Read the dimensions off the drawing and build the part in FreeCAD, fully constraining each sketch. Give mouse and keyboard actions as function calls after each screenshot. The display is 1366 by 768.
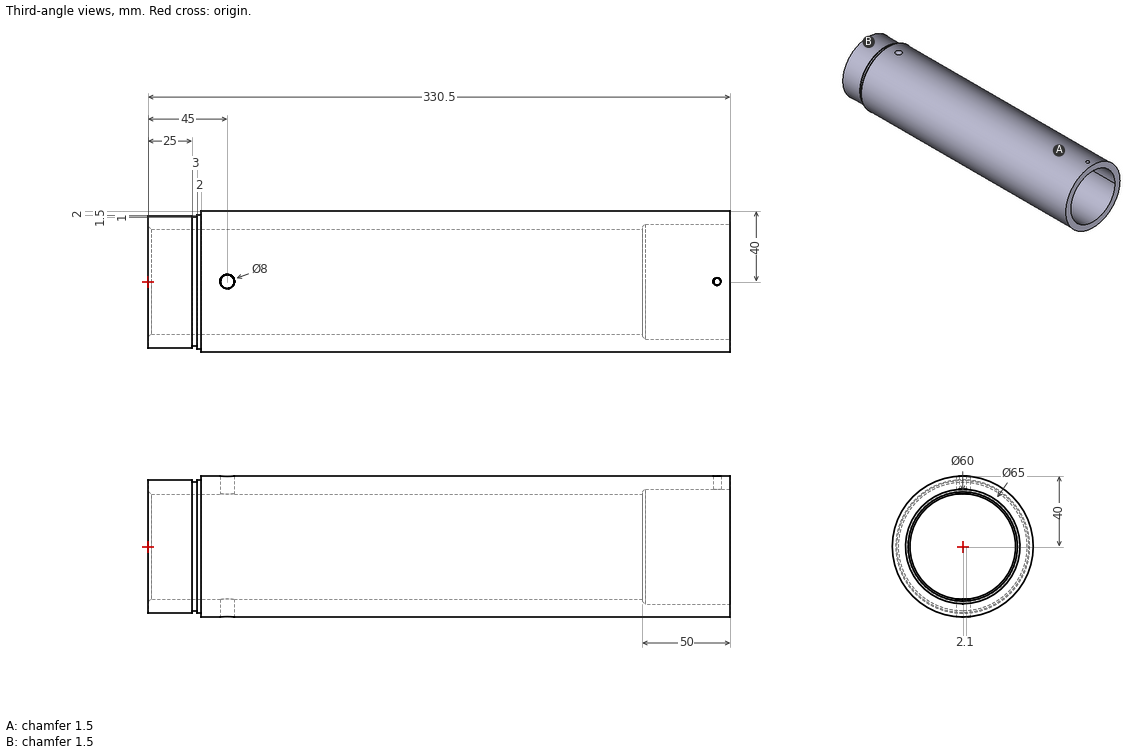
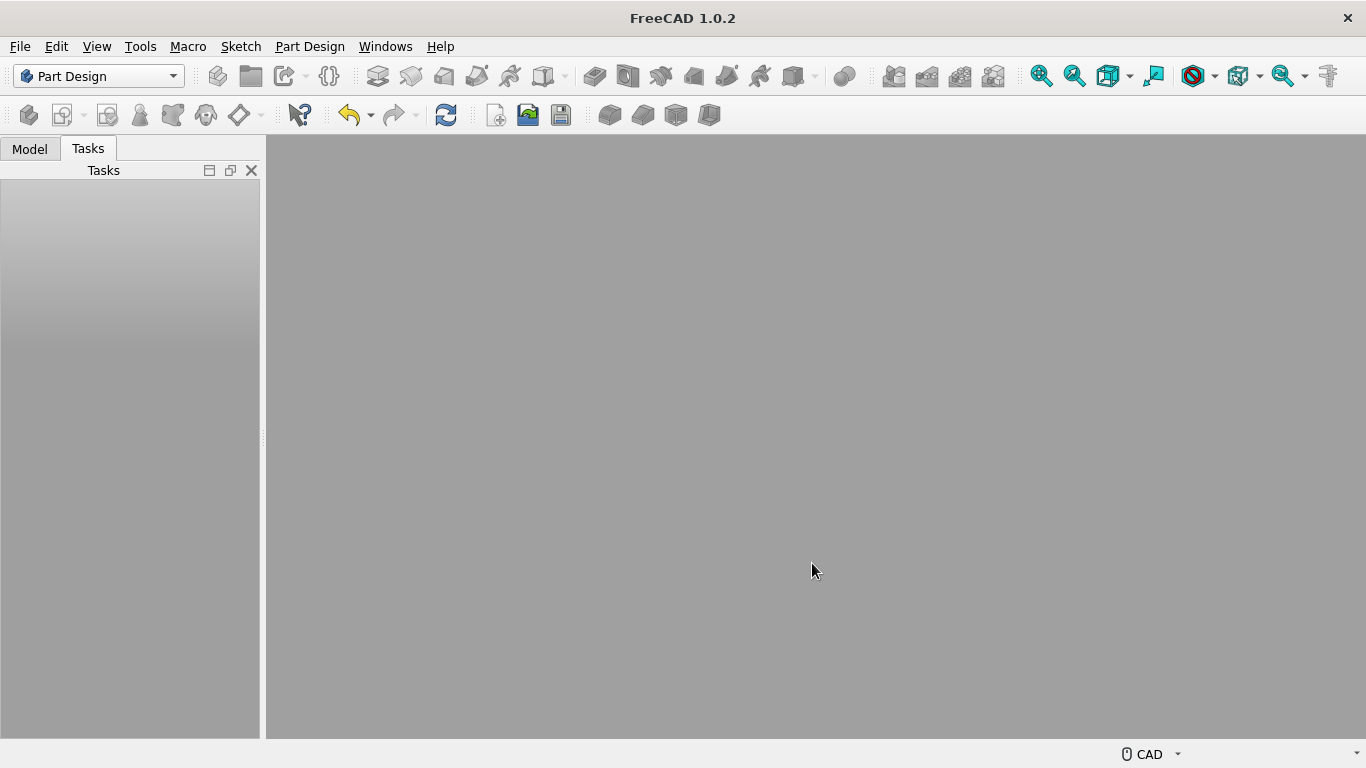
click(495, 116)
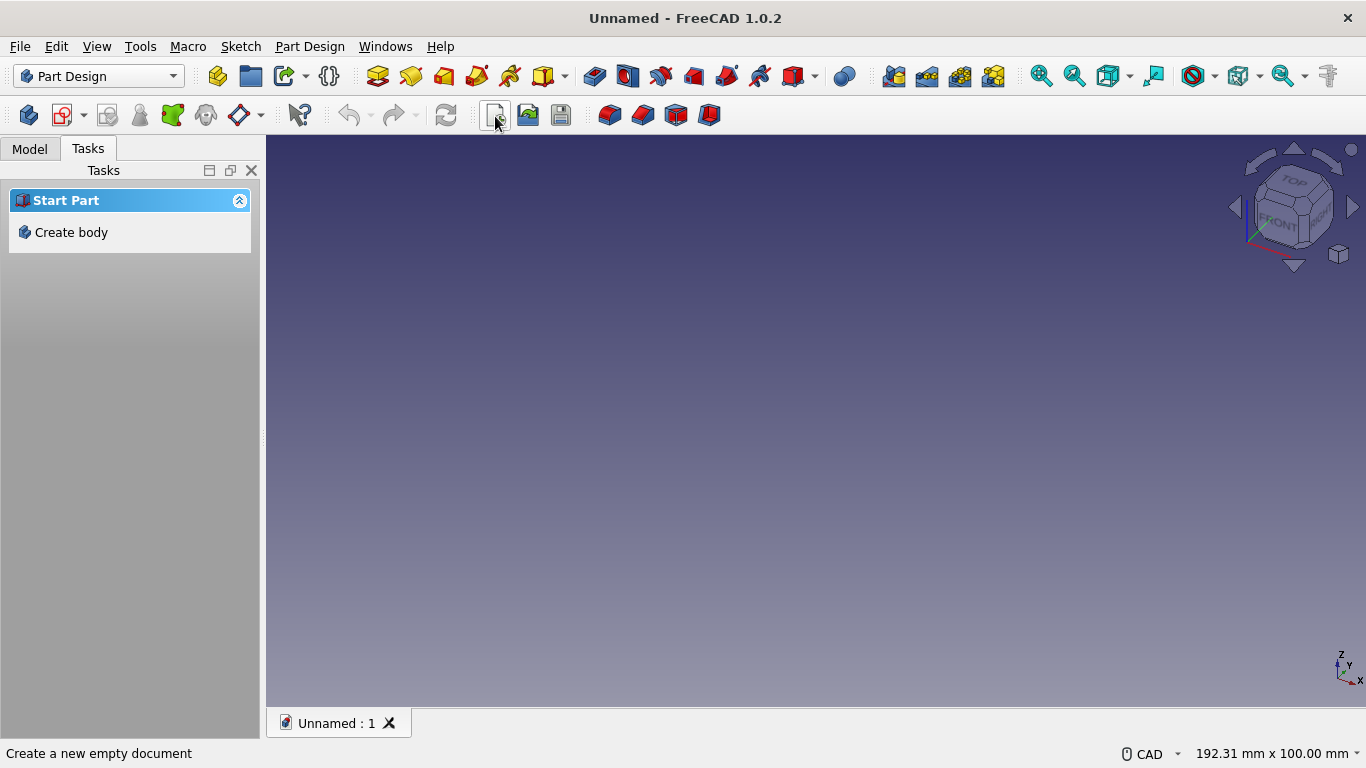
click(62, 116)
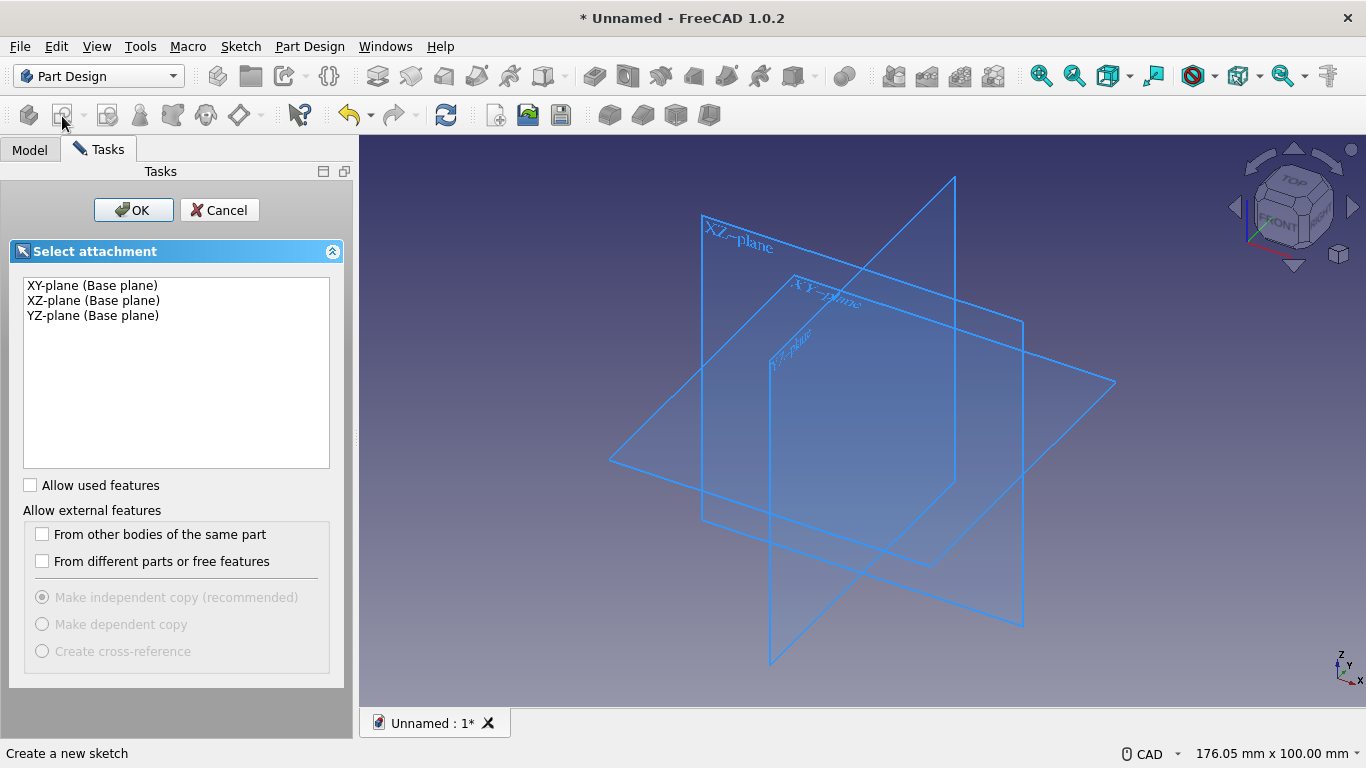
click(84, 286)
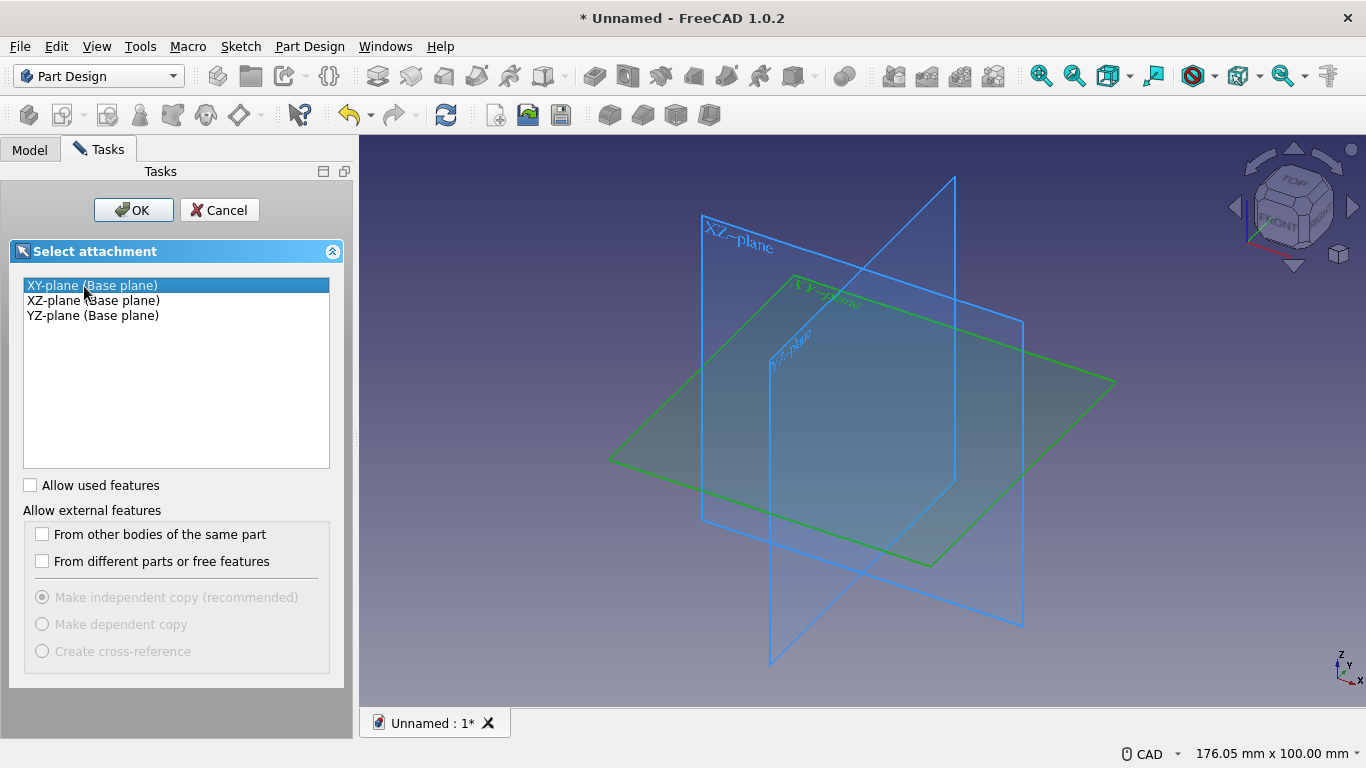
click(134, 210)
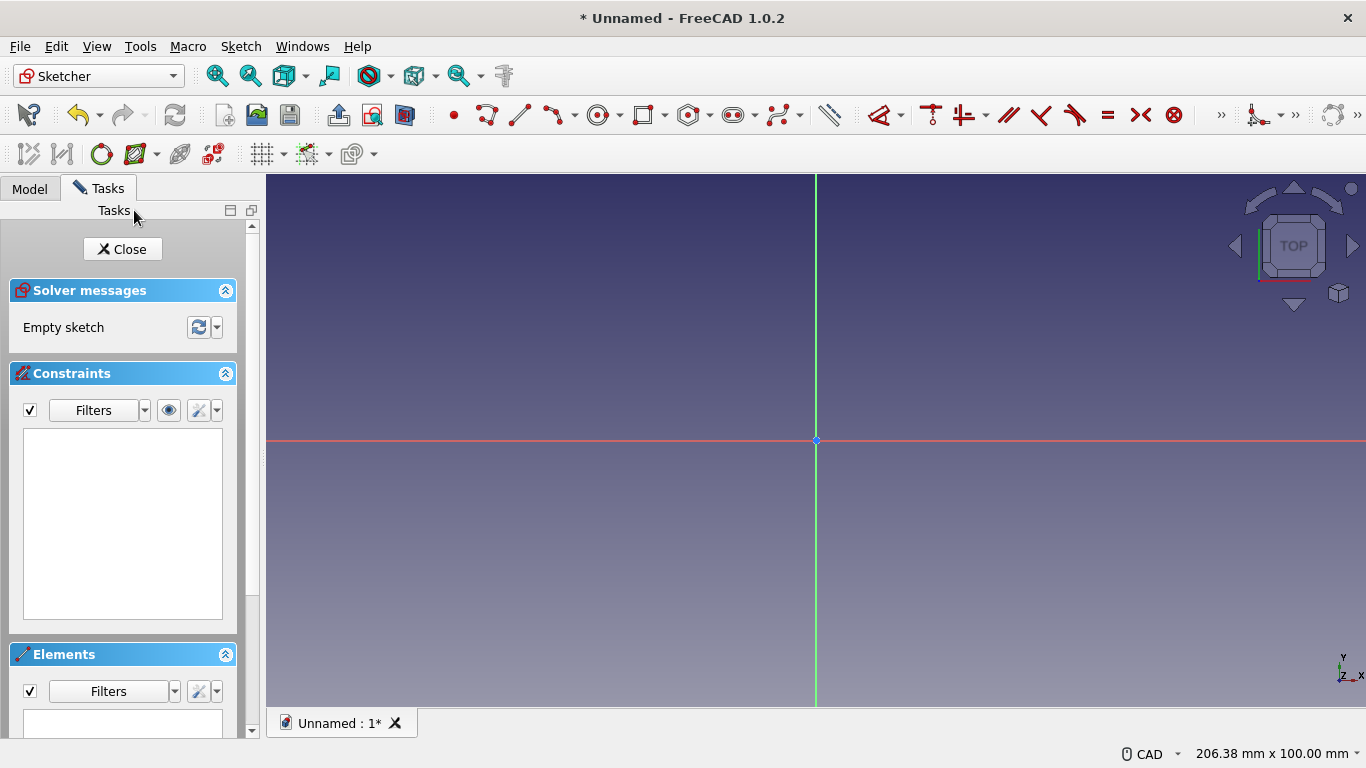
scroll(294, 503, down, 5)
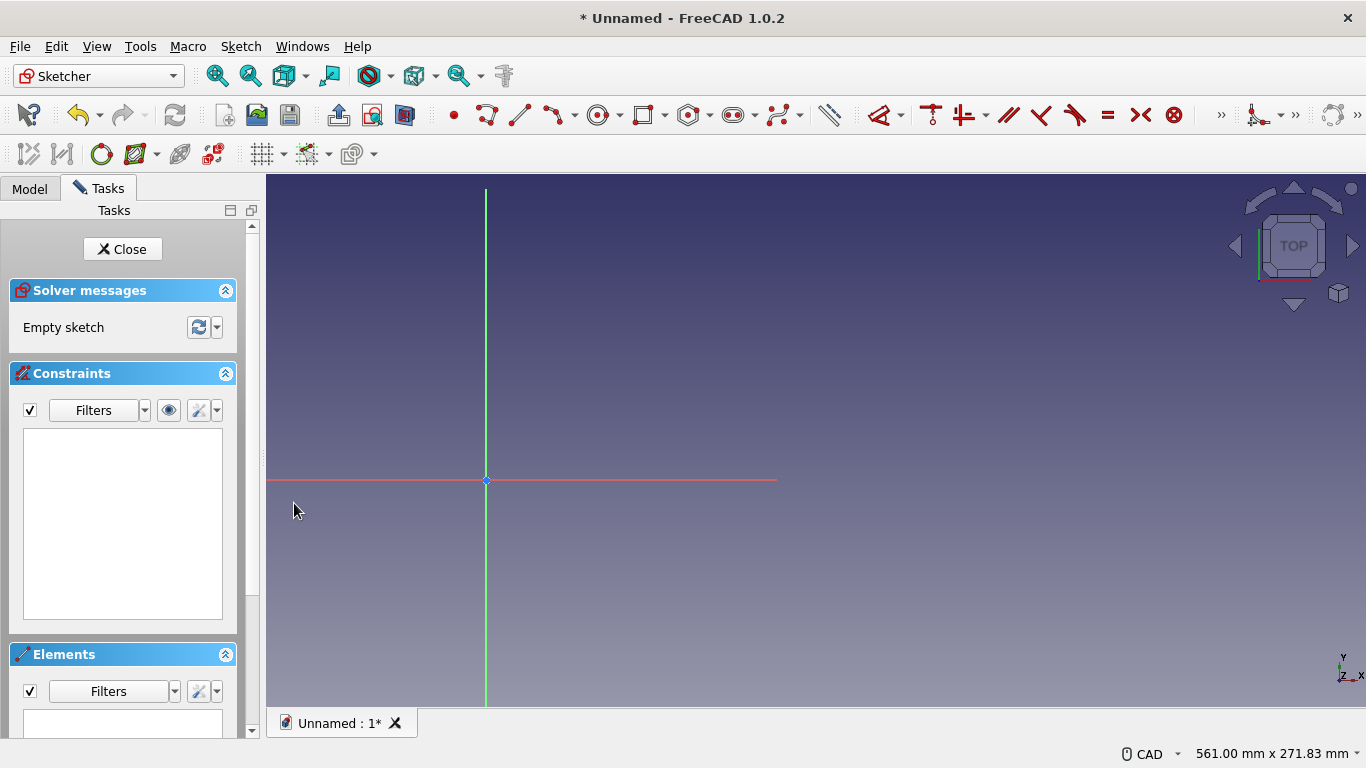
click(487, 116)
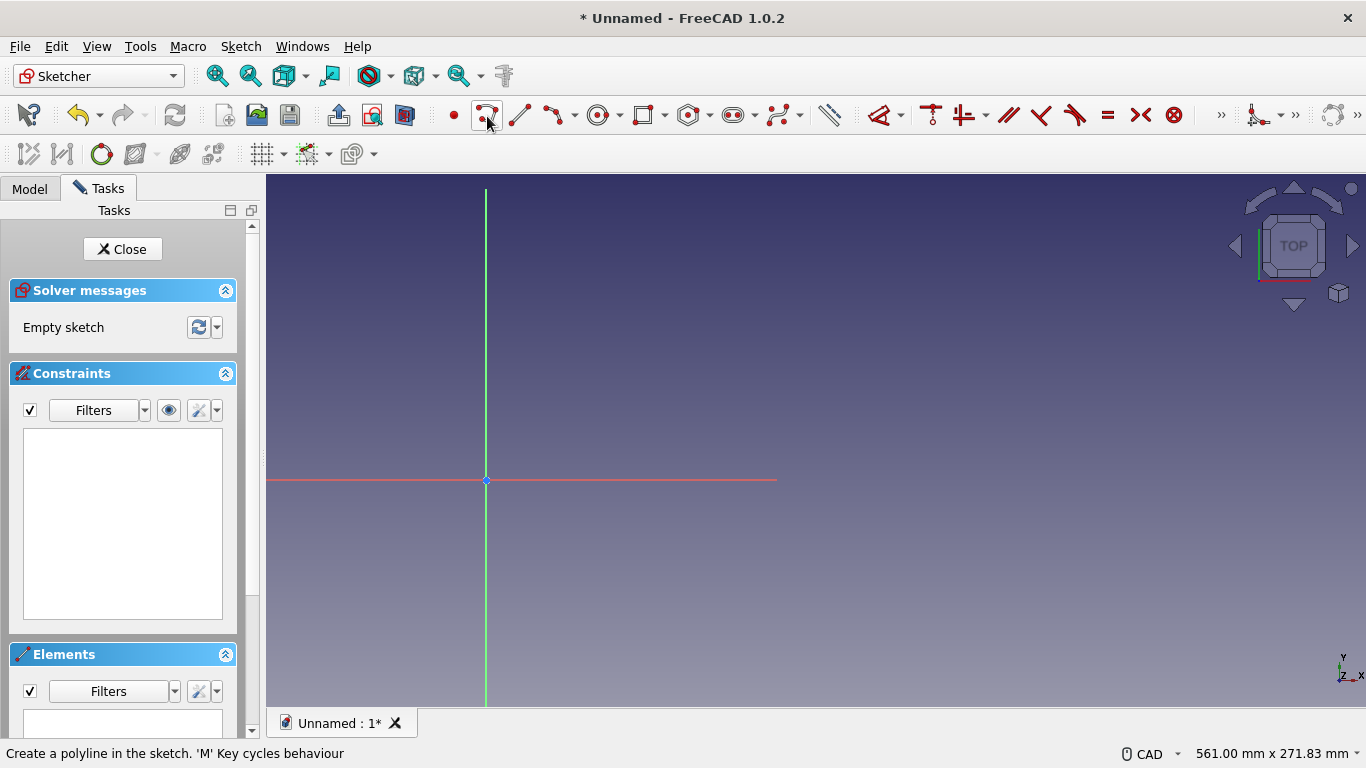
click(486, 480)
click(1134, 471)
click(1134, 402)
click(545, 402)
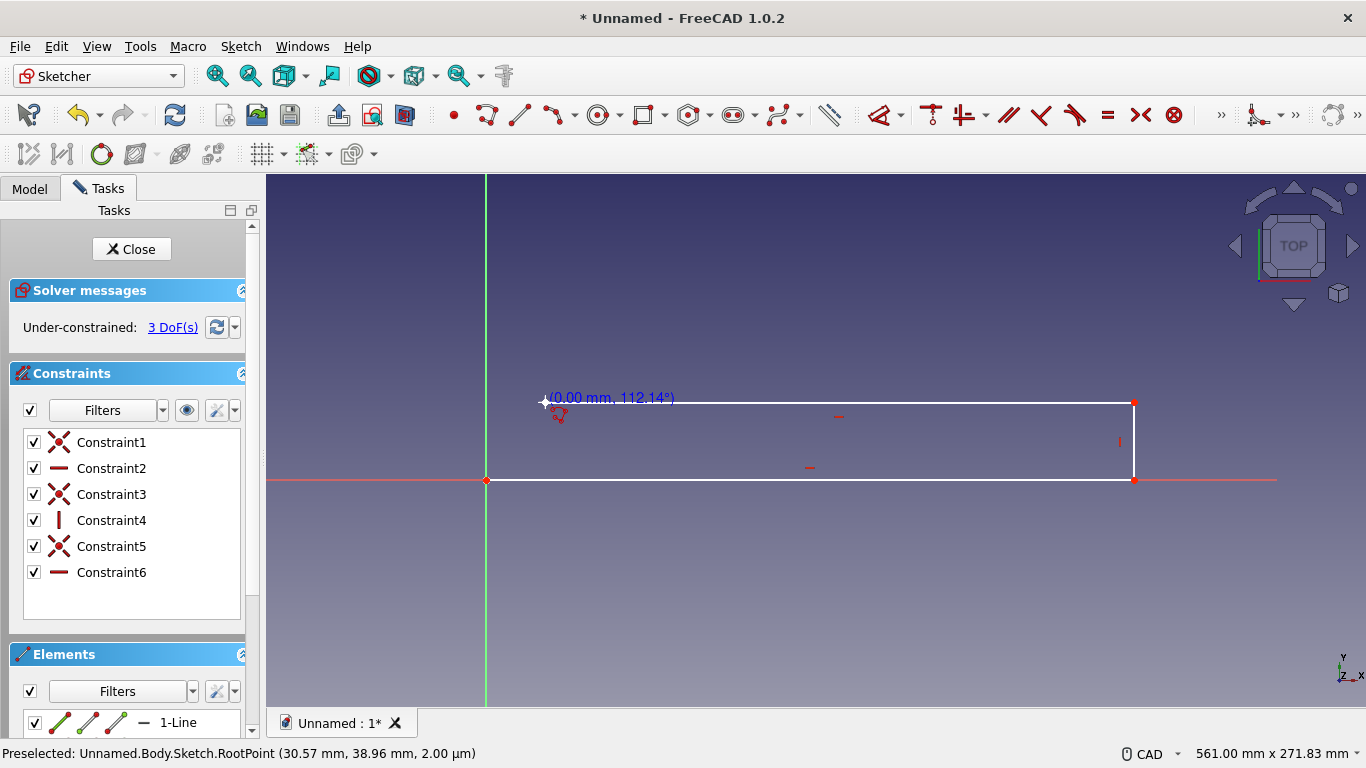
scroll(545, 406, up, 7)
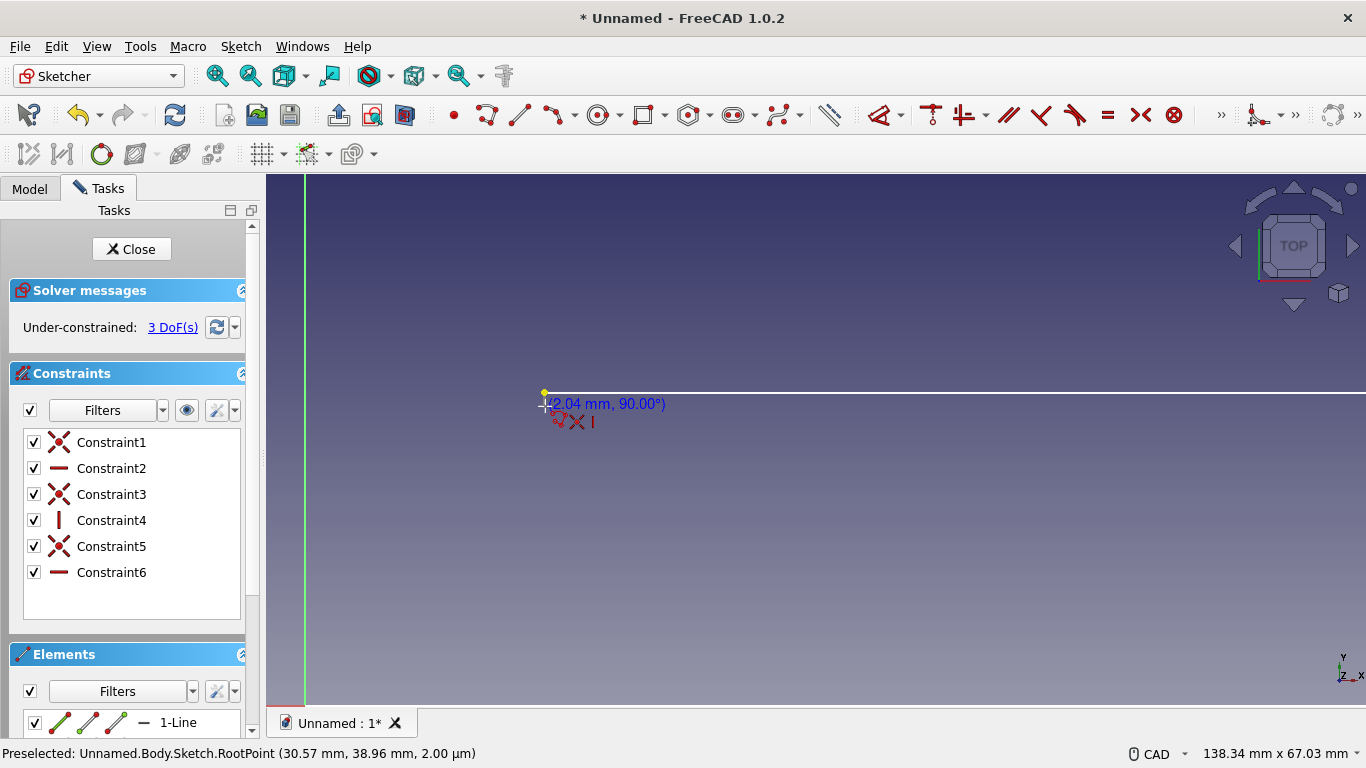
click(544, 404)
click(528, 404)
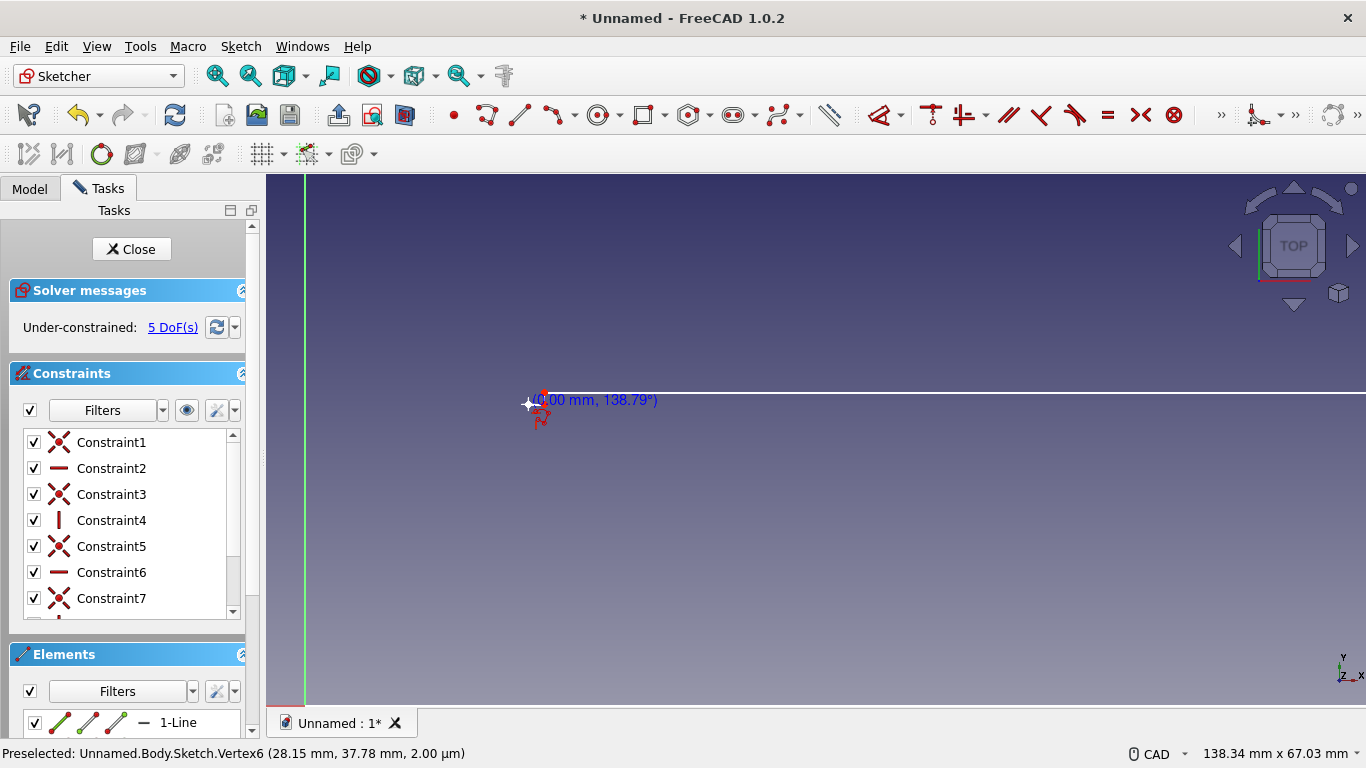
scroll(528, 416, up, 2)